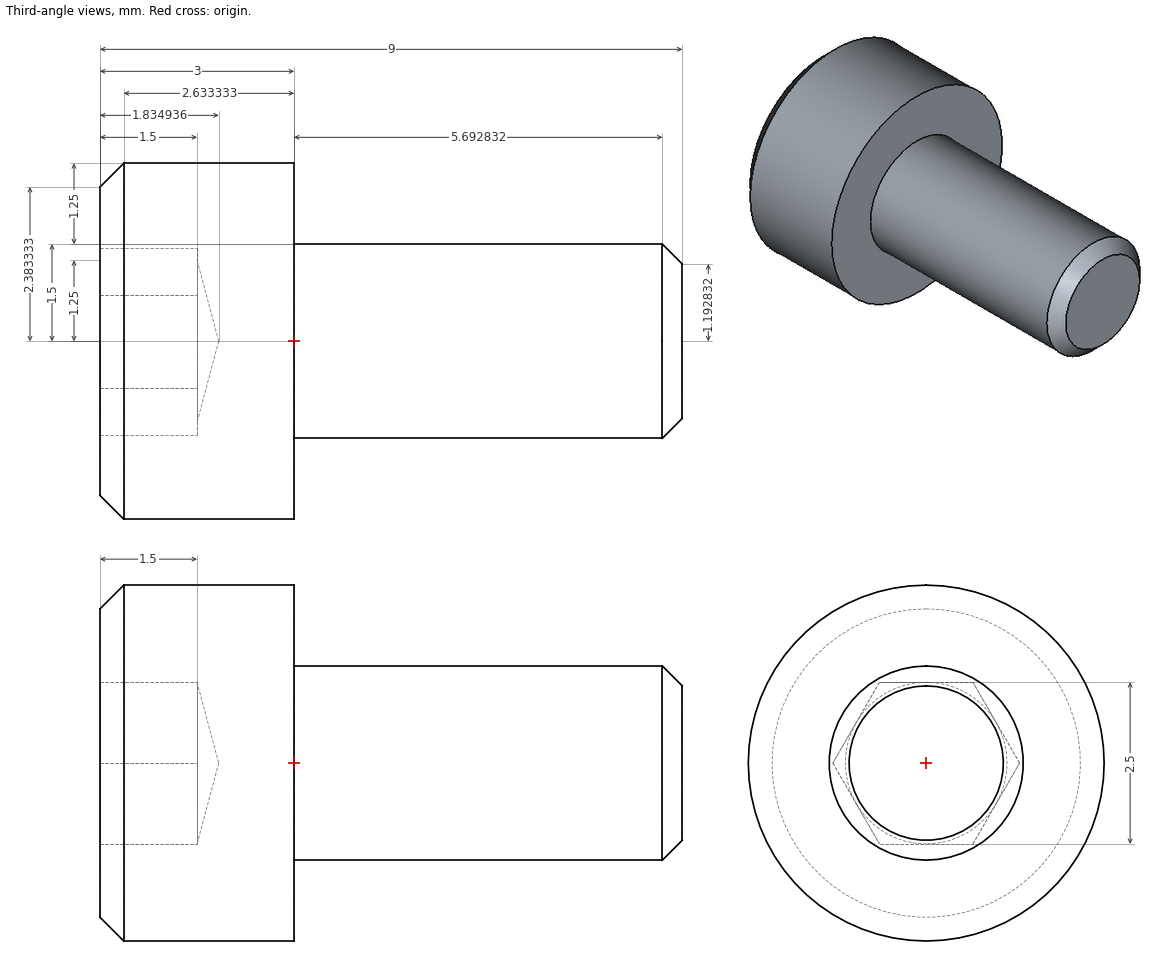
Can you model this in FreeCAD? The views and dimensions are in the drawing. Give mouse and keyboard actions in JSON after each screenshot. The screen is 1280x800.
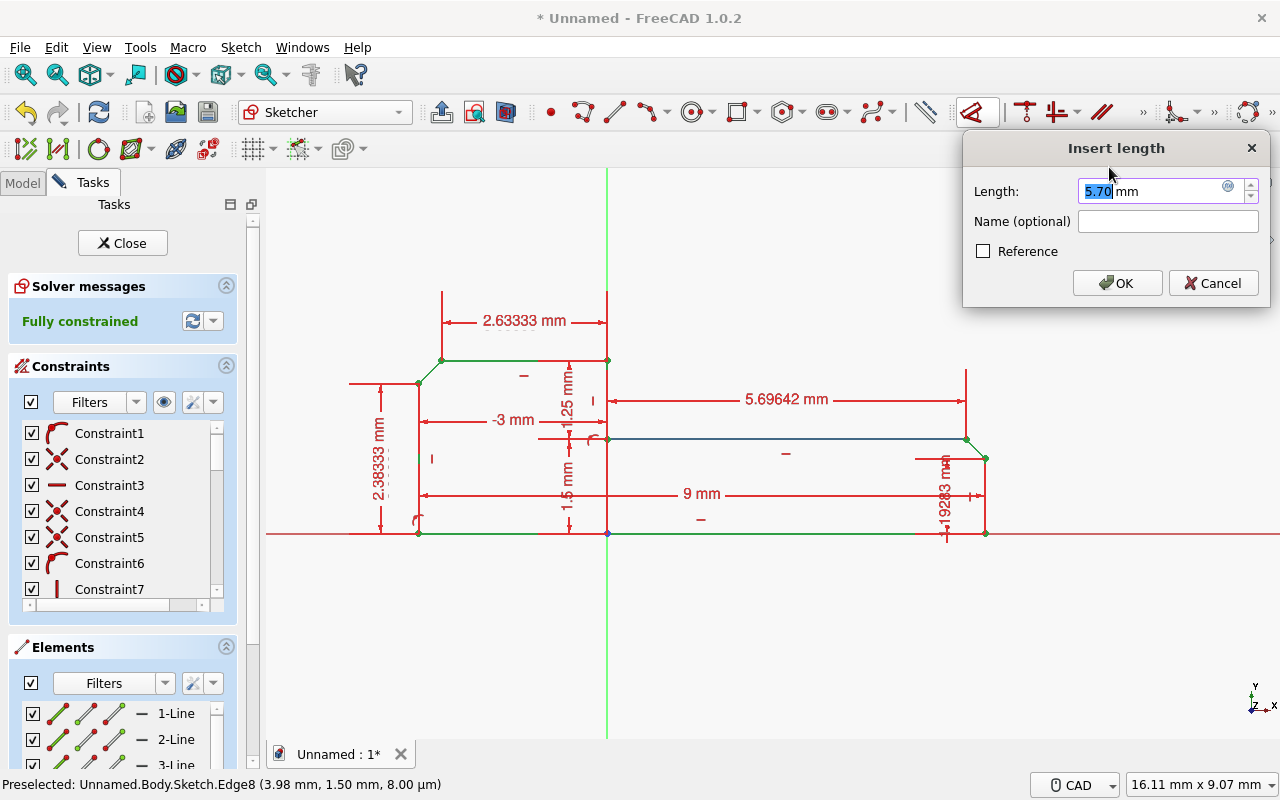
{"action": "type", "text": "5.692832"}
{"action": "key", "text": "Return"}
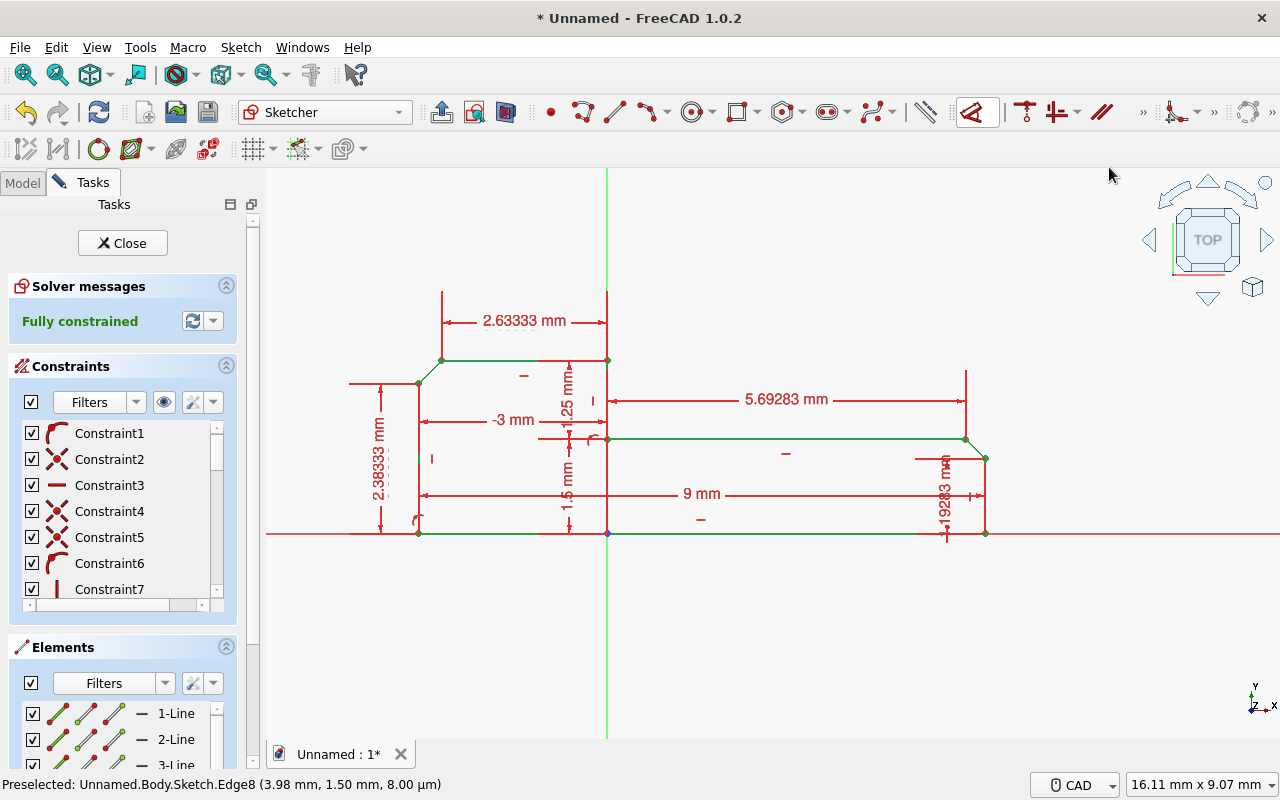
{"action": "left_click", "coordinate": [123, 243]}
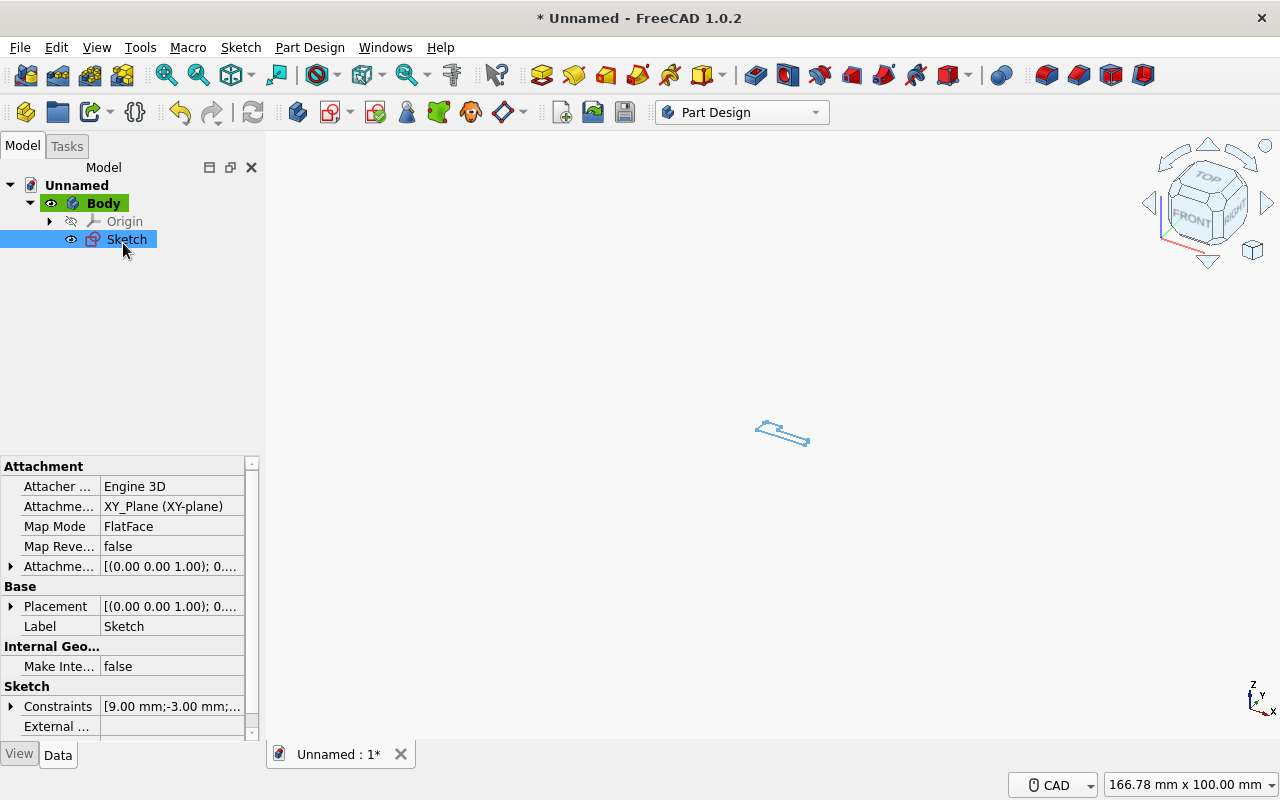
{"action": "left_click", "coordinate": [574, 76]}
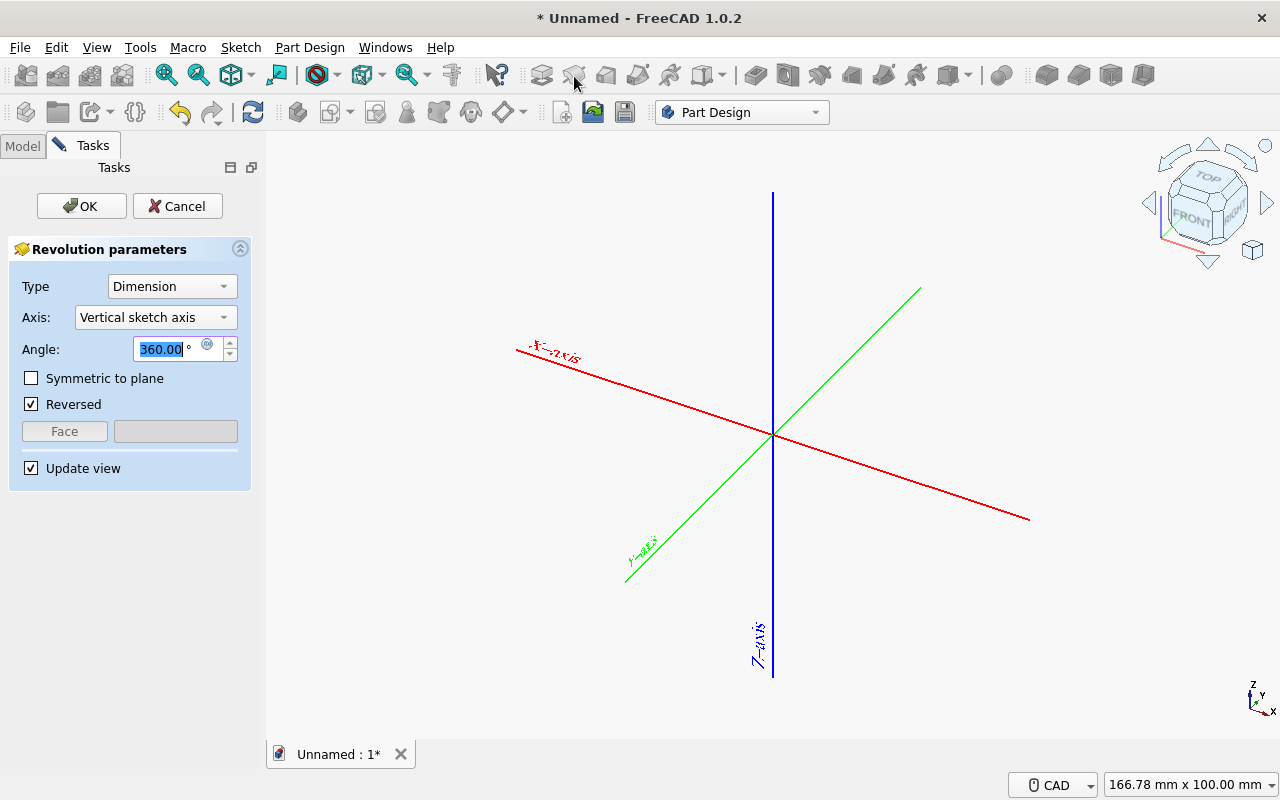
{"action": "left_click", "coordinate": [156, 318]}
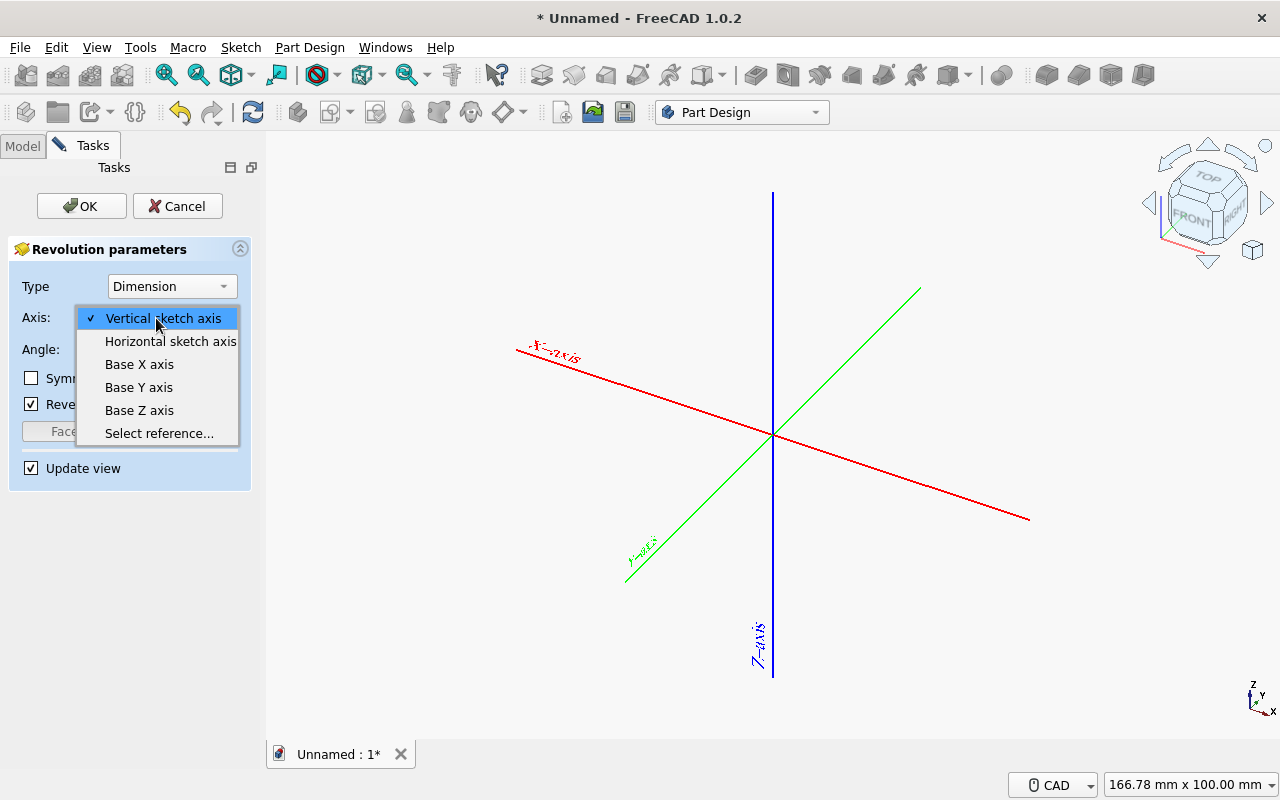
{"action": "left_click", "coordinate": [156, 342]}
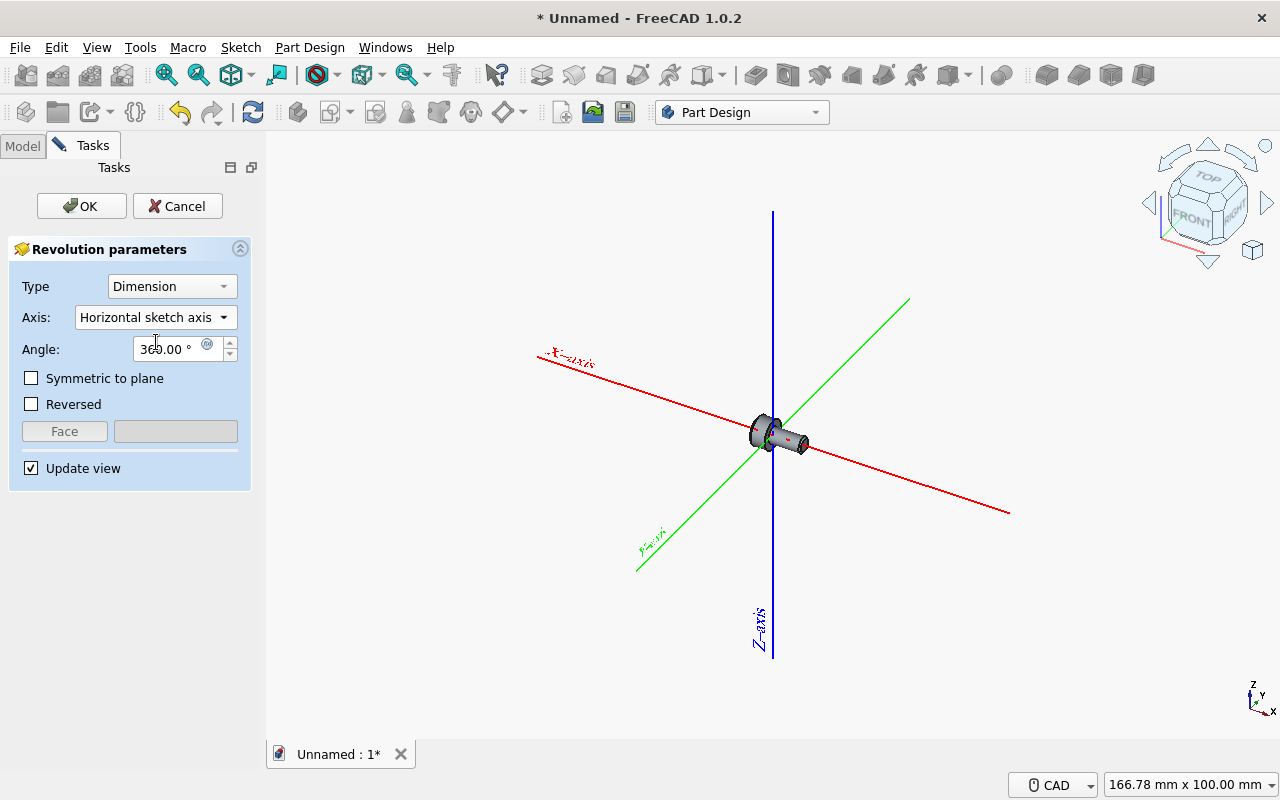
{"action": "left_click", "coordinate": [82, 206]}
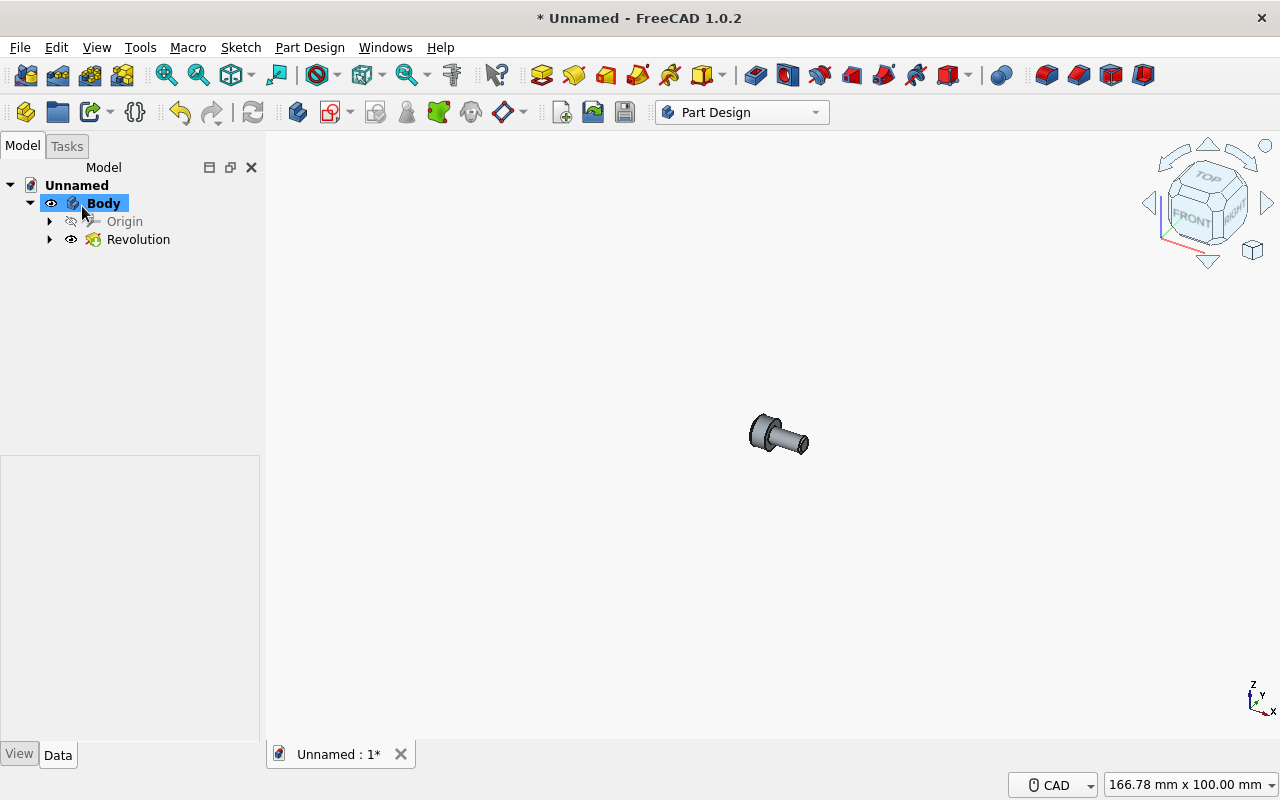
{"action": "left_click", "coordinate": [168, 76]}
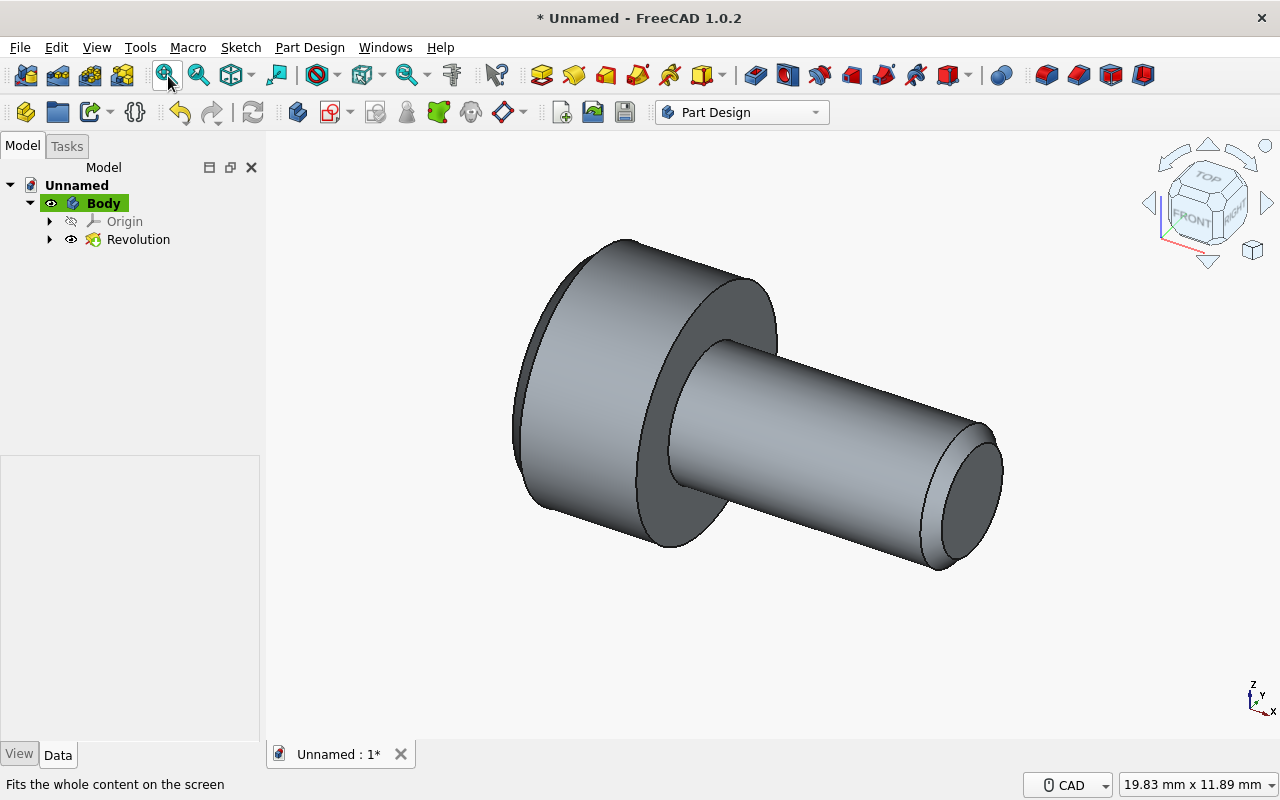
{"action": "left_click", "coordinate": [330, 112]}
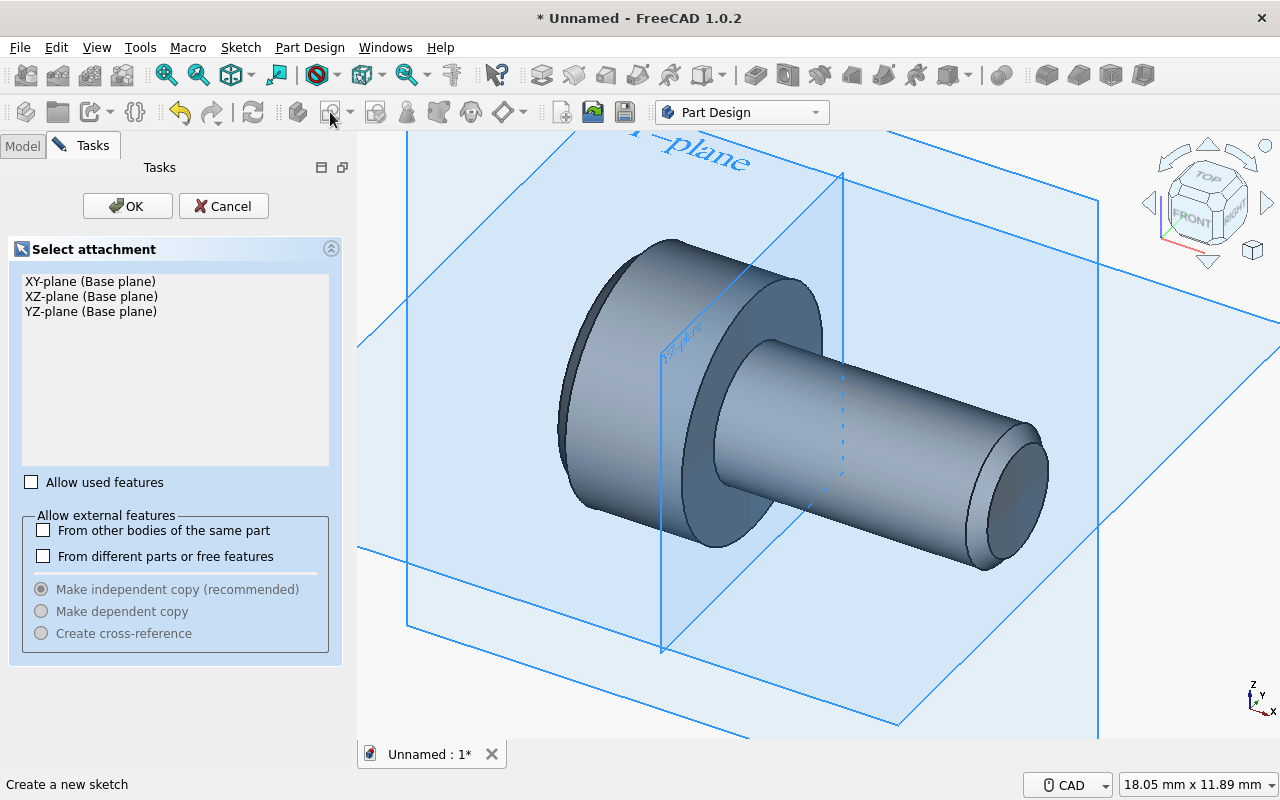
{"action": "left_click", "coordinate": [82, 282]}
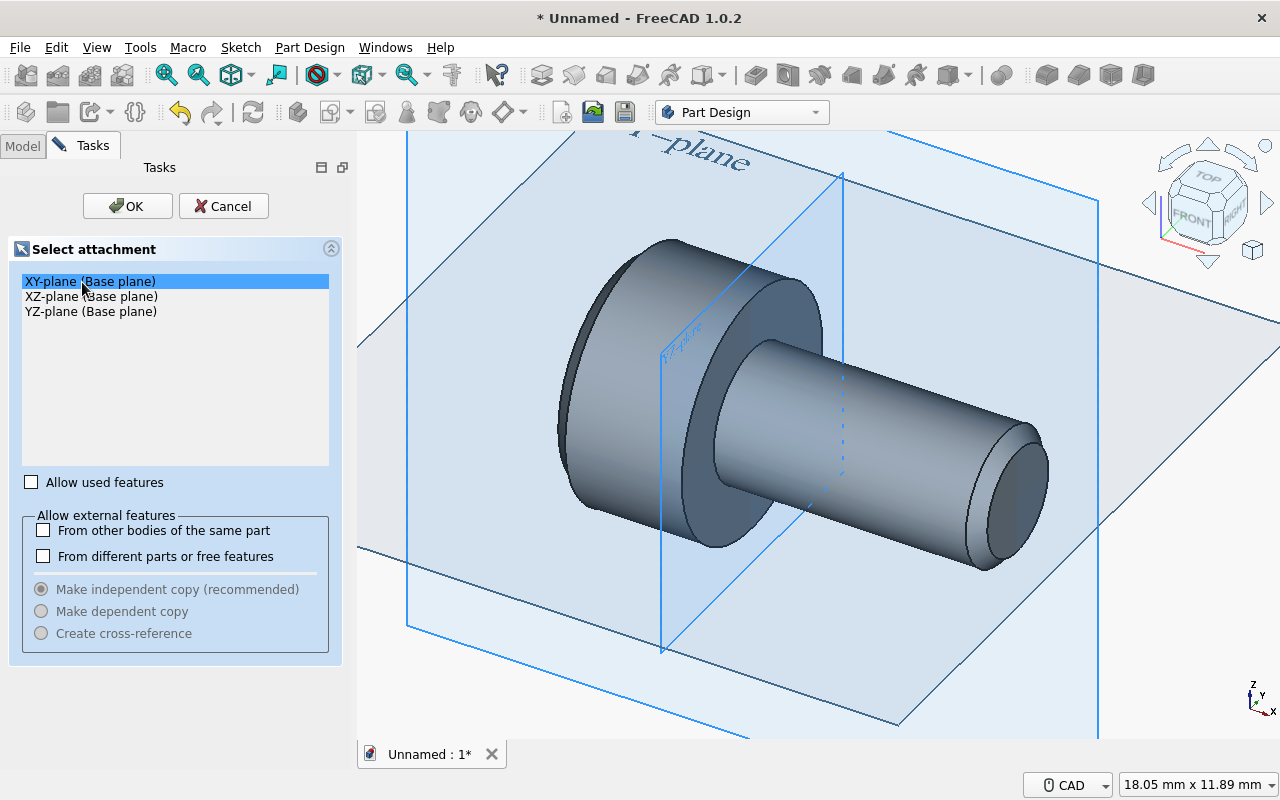
{"action": "left_click", "coordinate": [128, 206]}